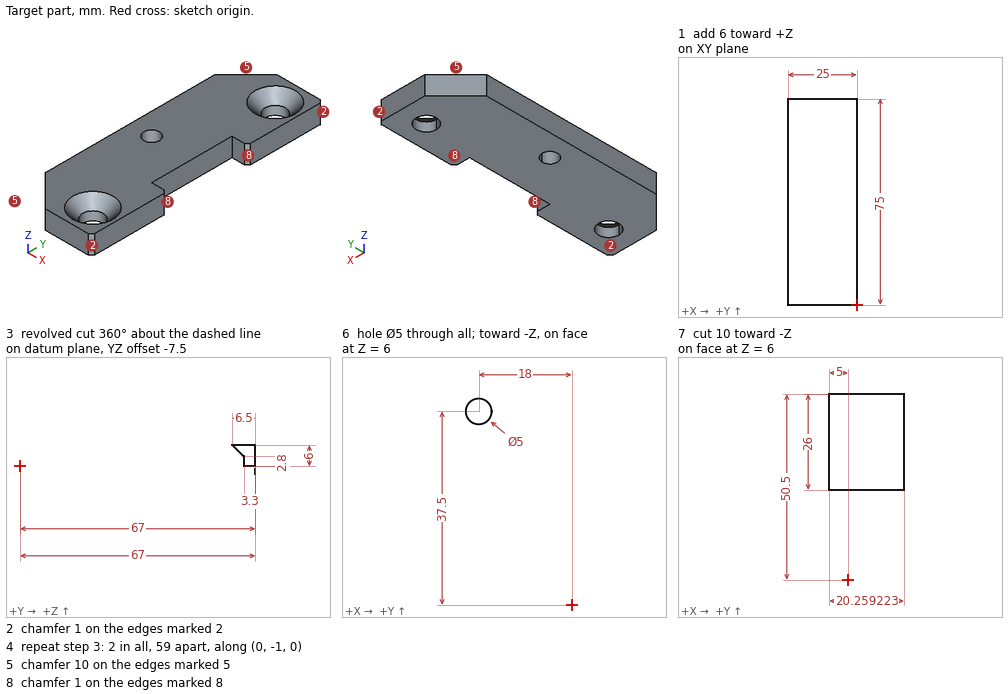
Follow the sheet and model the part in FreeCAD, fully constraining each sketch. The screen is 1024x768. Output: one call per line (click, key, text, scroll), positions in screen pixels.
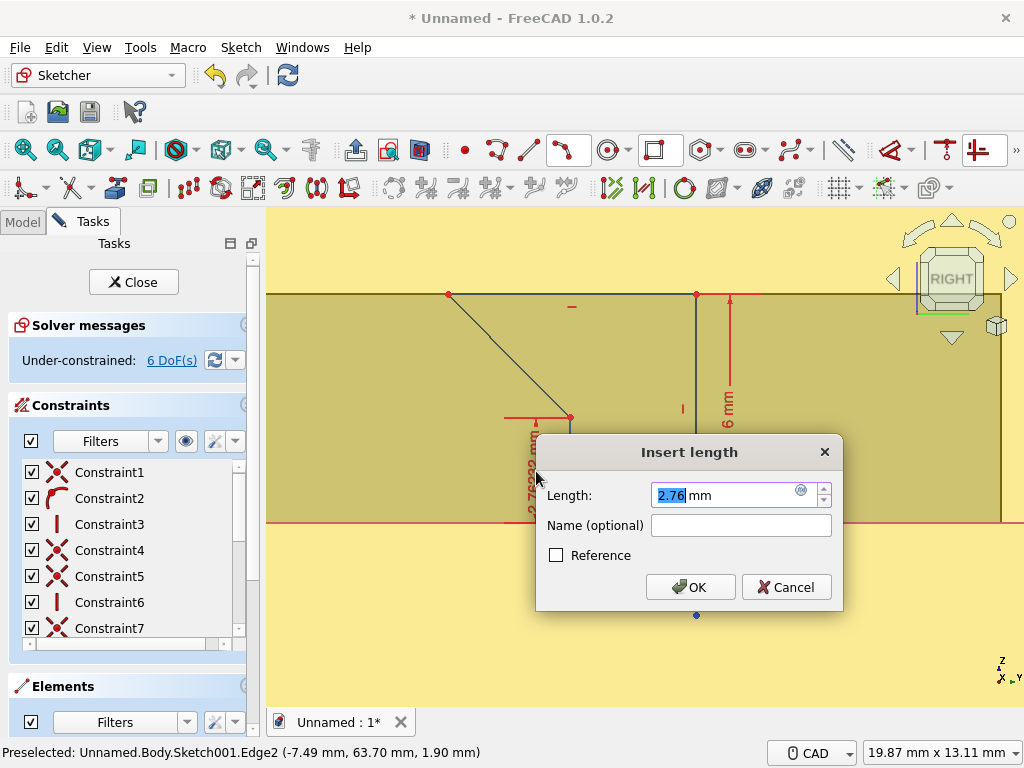
text(2.8)
key(Return)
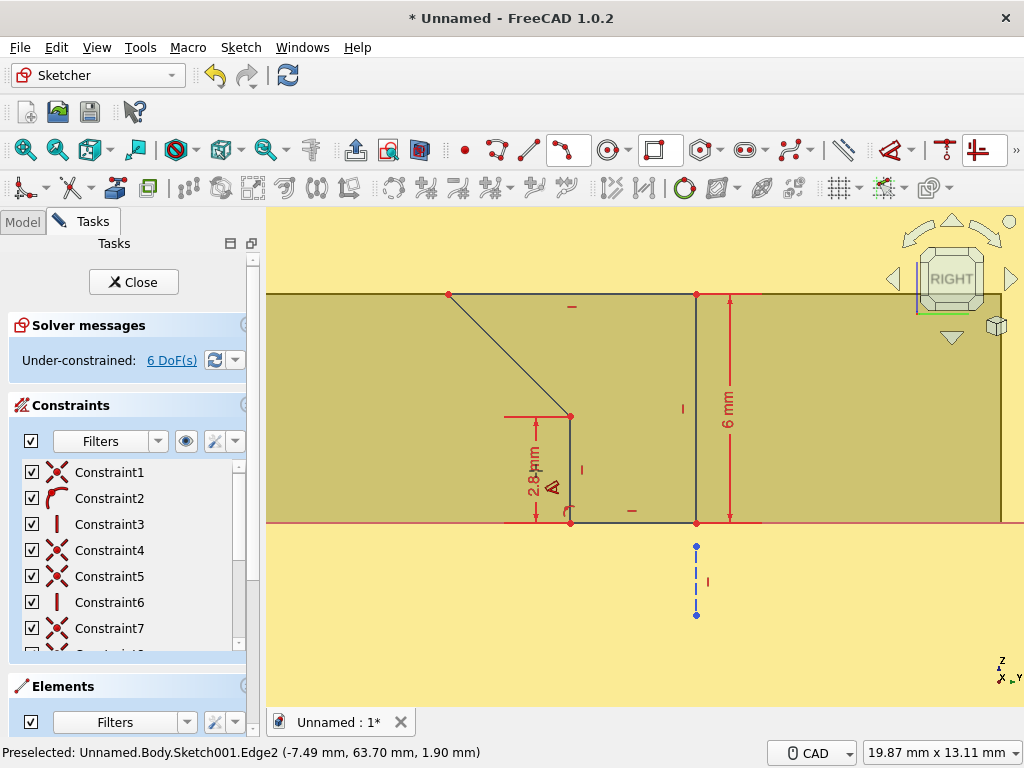
click(608, 523)
click(633, 557)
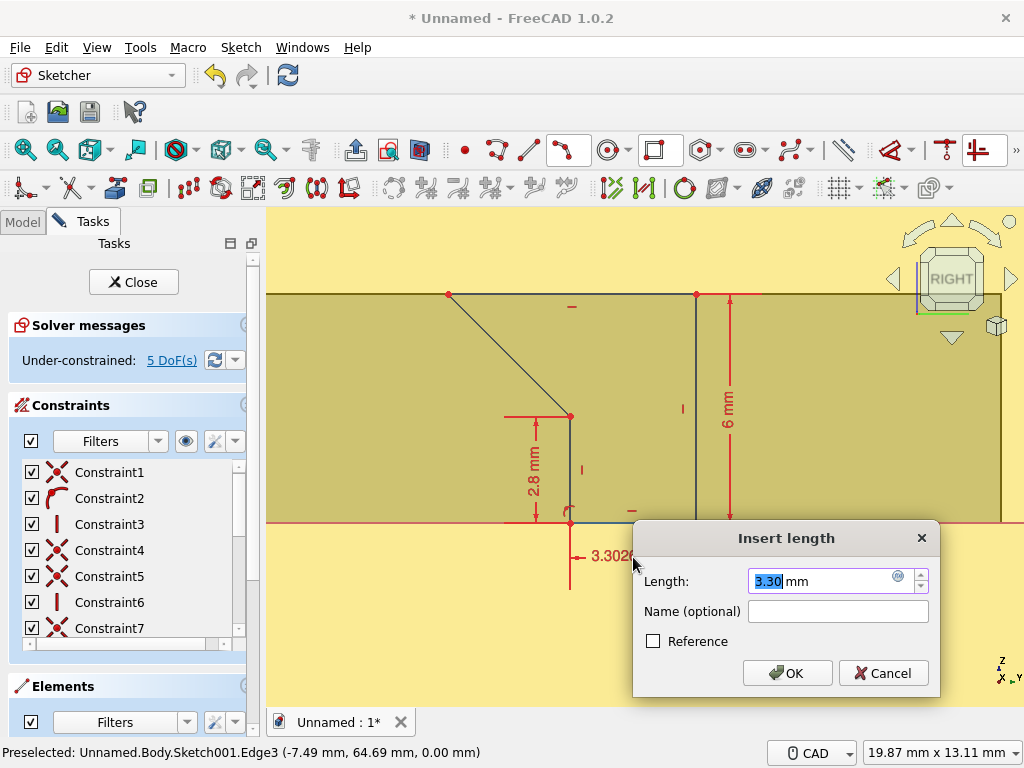
text(3.3)
key(Return)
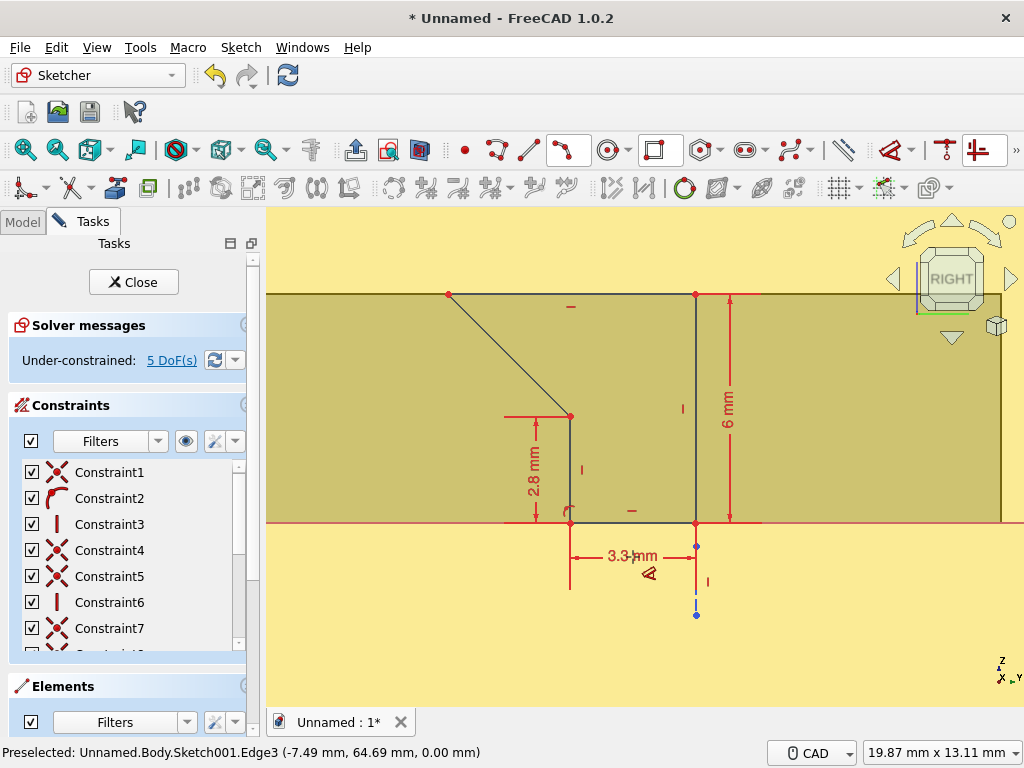
click(622, 294)
click(572, 260)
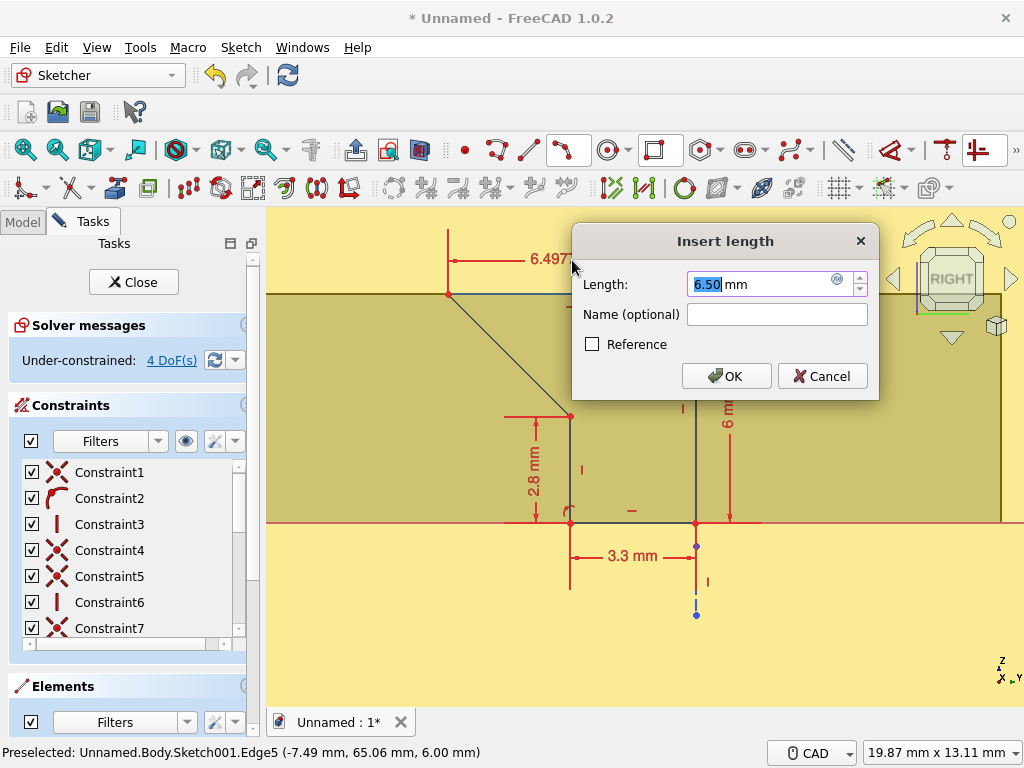
text(6.5)
key(Return)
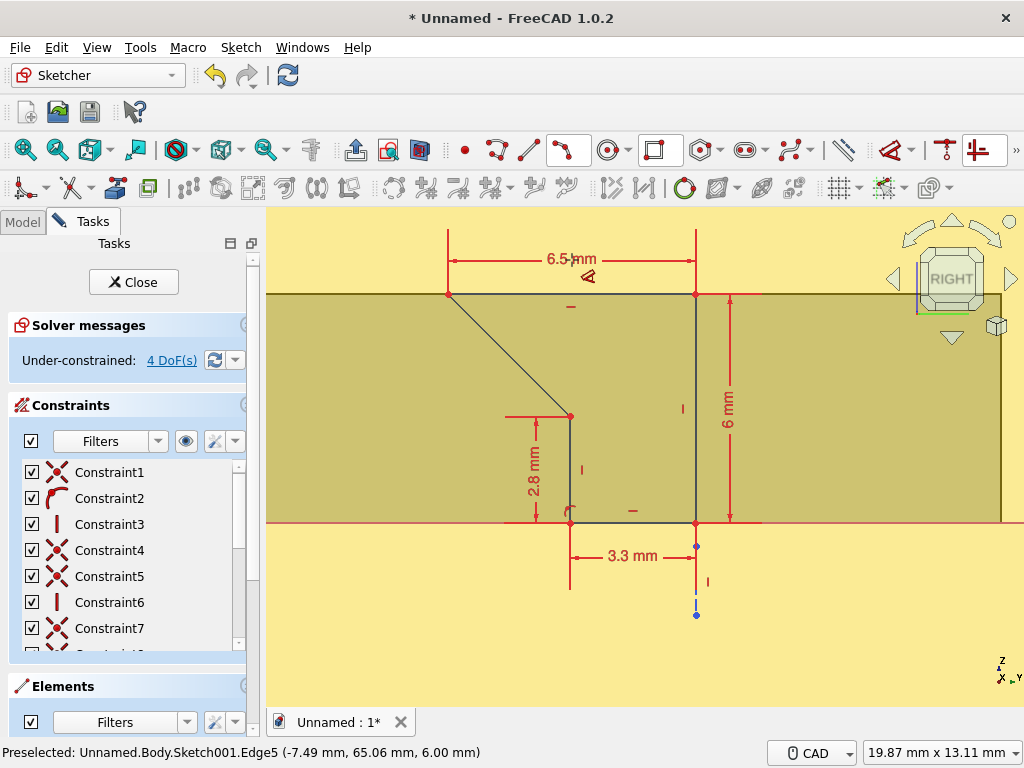
click(696, 523)
click(495, 557)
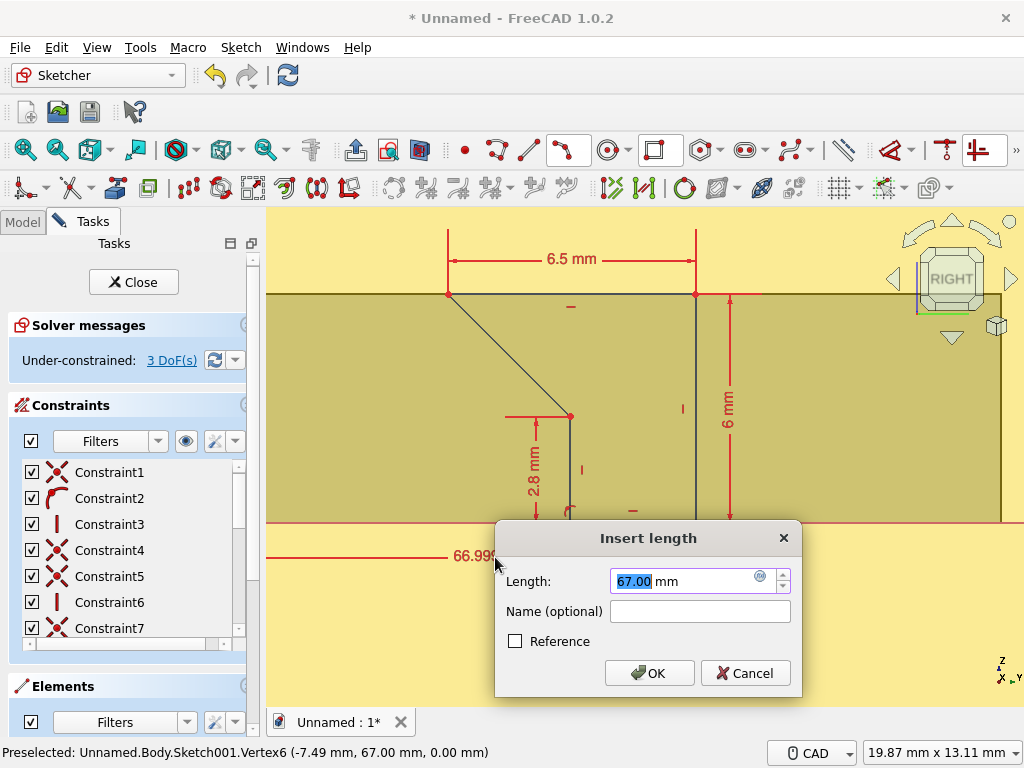
text(67)
key(Return)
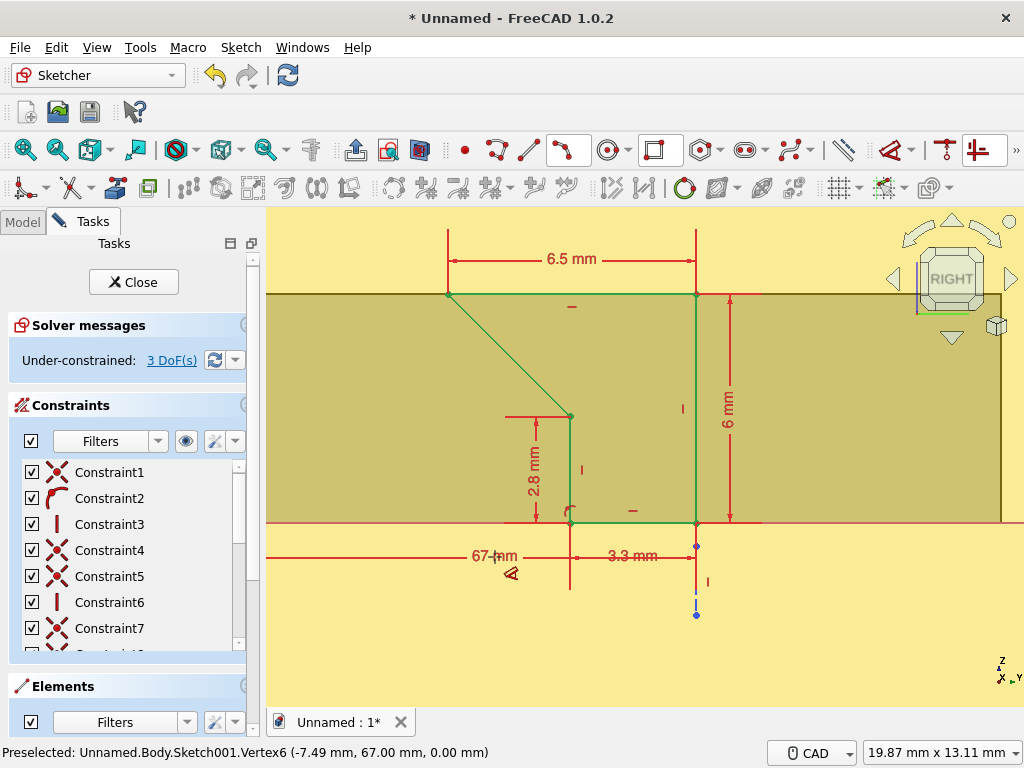
click(696, 547)
click(495, 581)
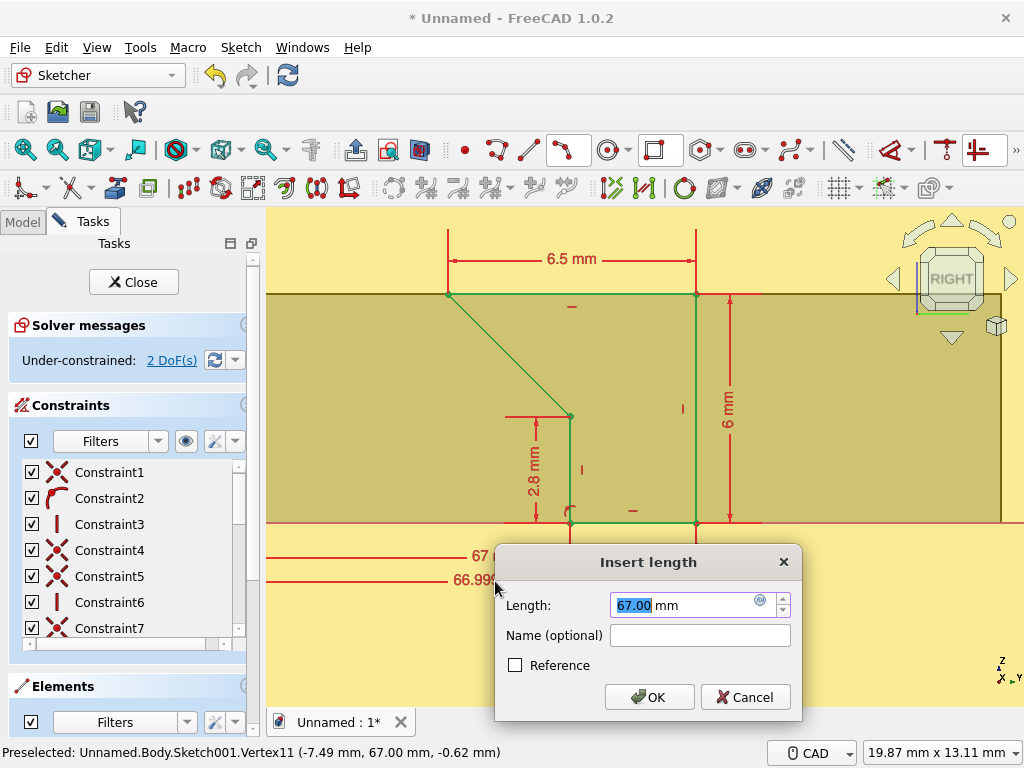
text(67)
key(Return)
key(Escape)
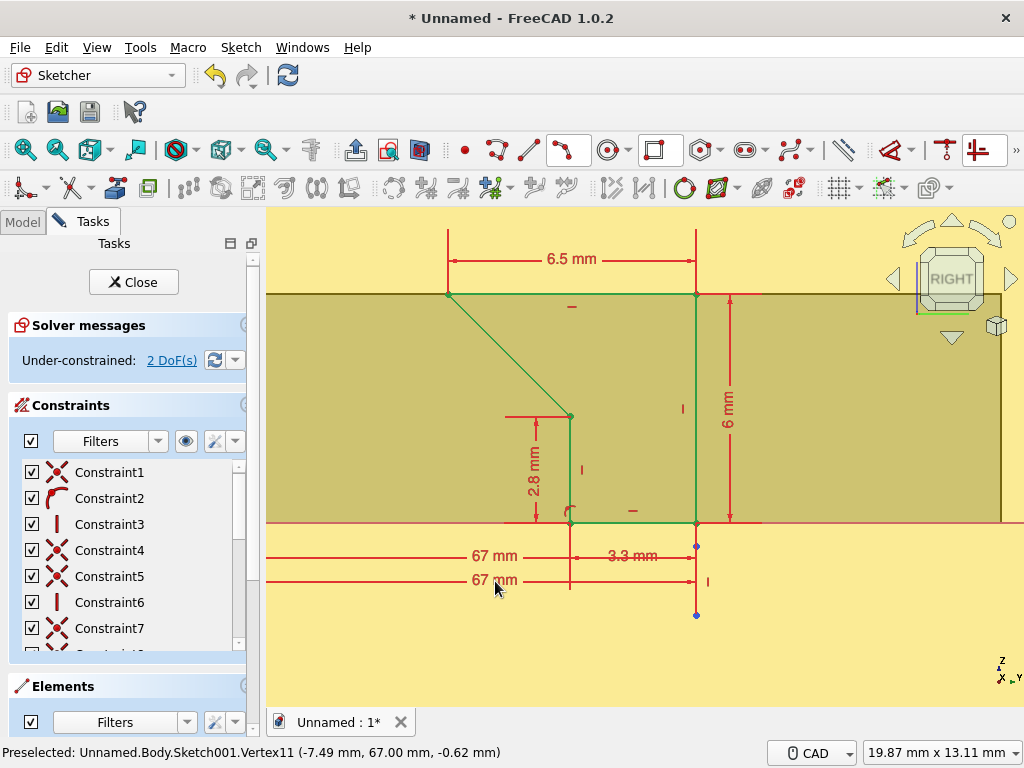
click(134, 282)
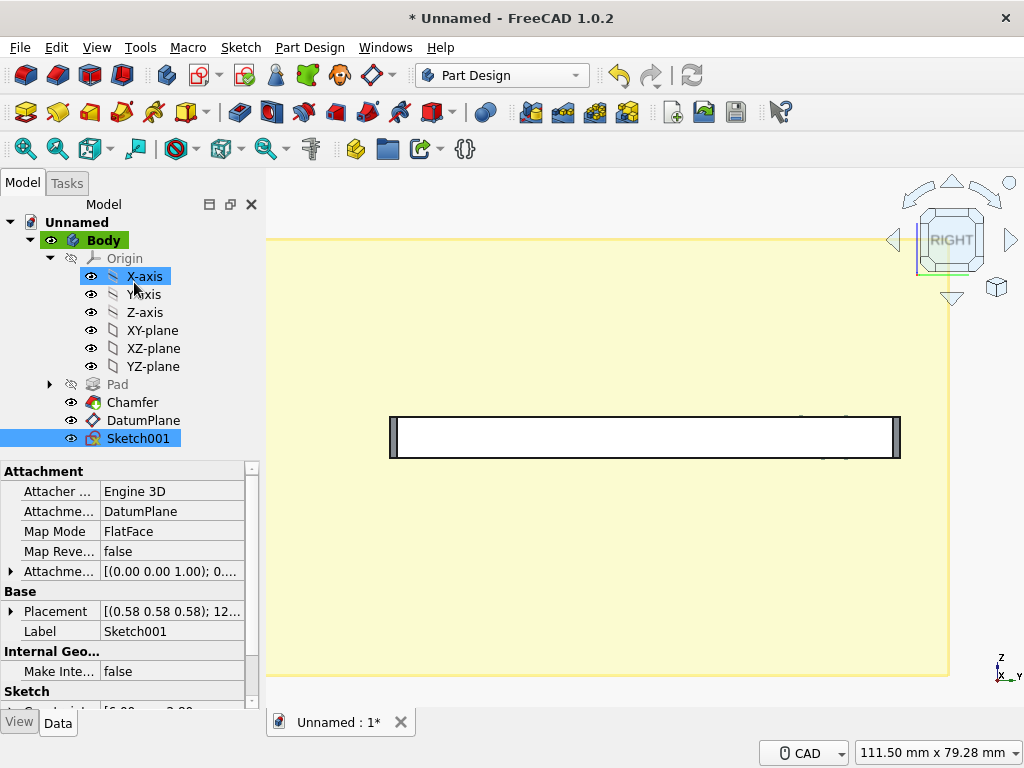
click(304, 112)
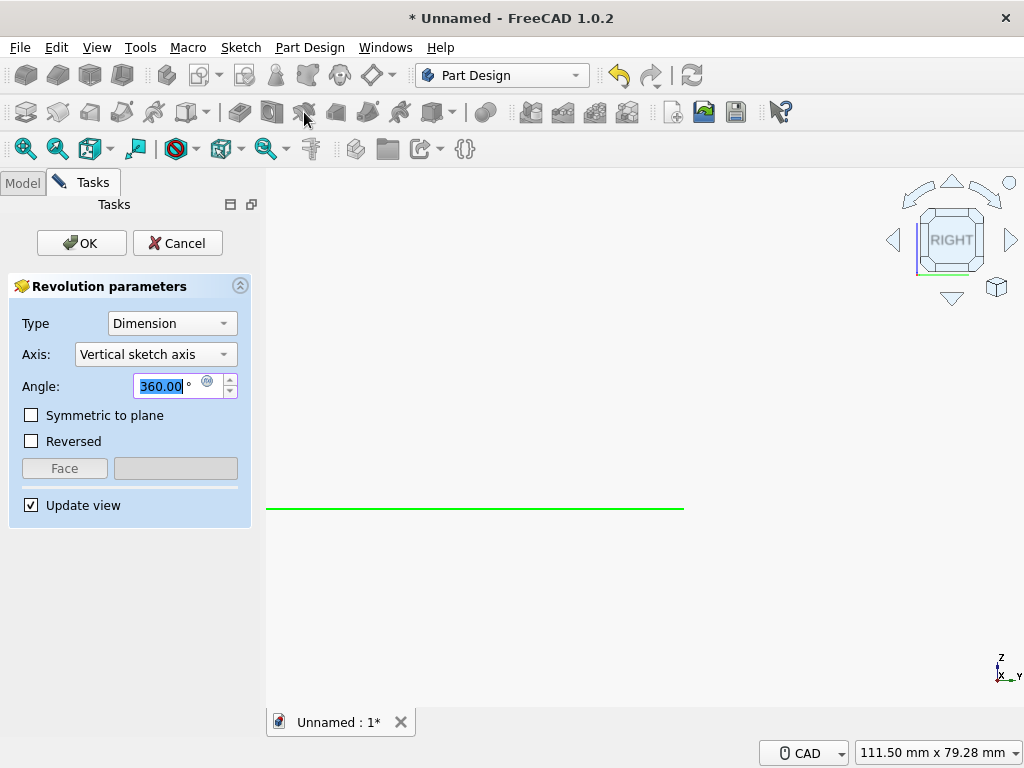
click(156, 354)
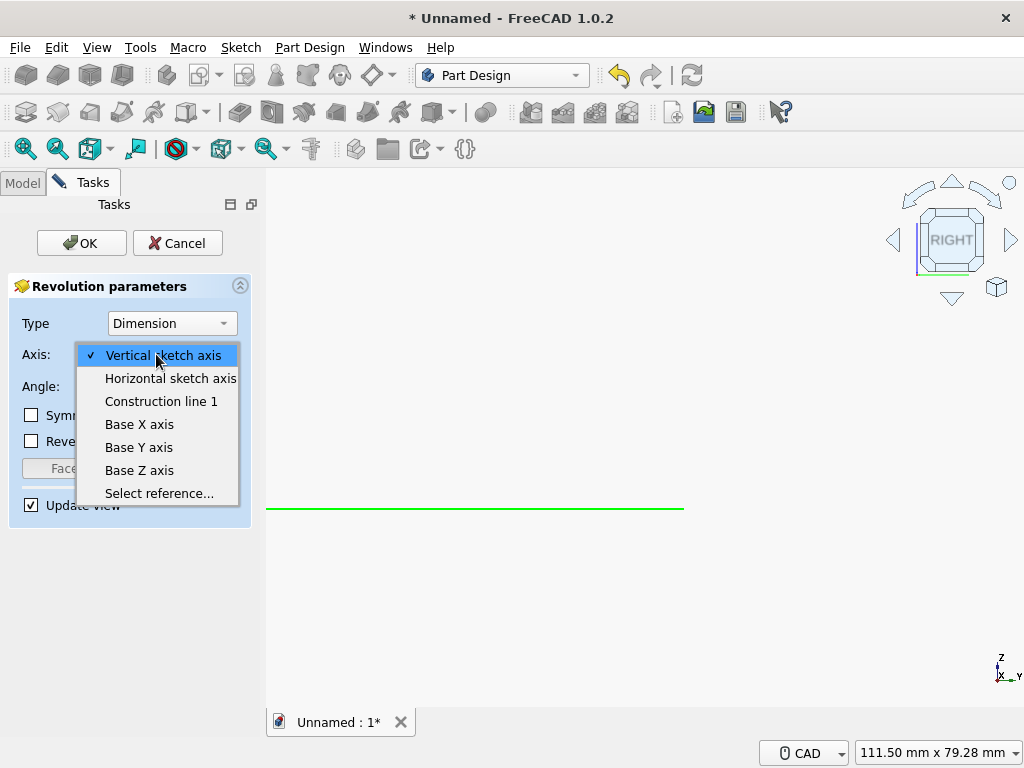
click(156, 402)